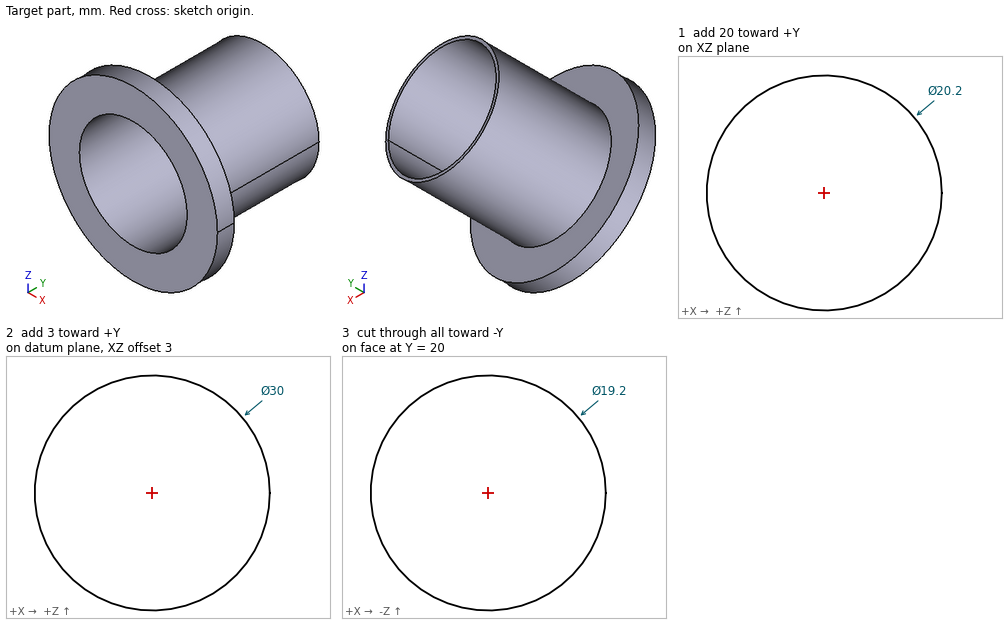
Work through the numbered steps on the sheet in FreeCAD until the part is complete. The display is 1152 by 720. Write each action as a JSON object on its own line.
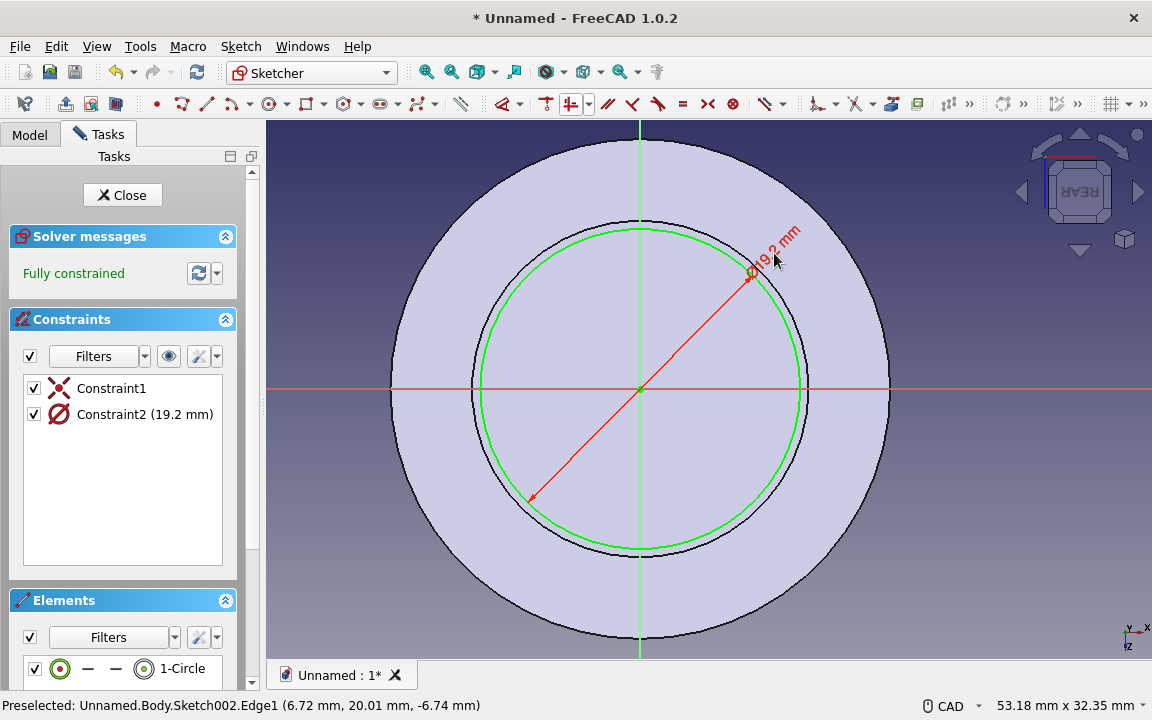
{"action": "left_click", "coordinate": [123, 195]}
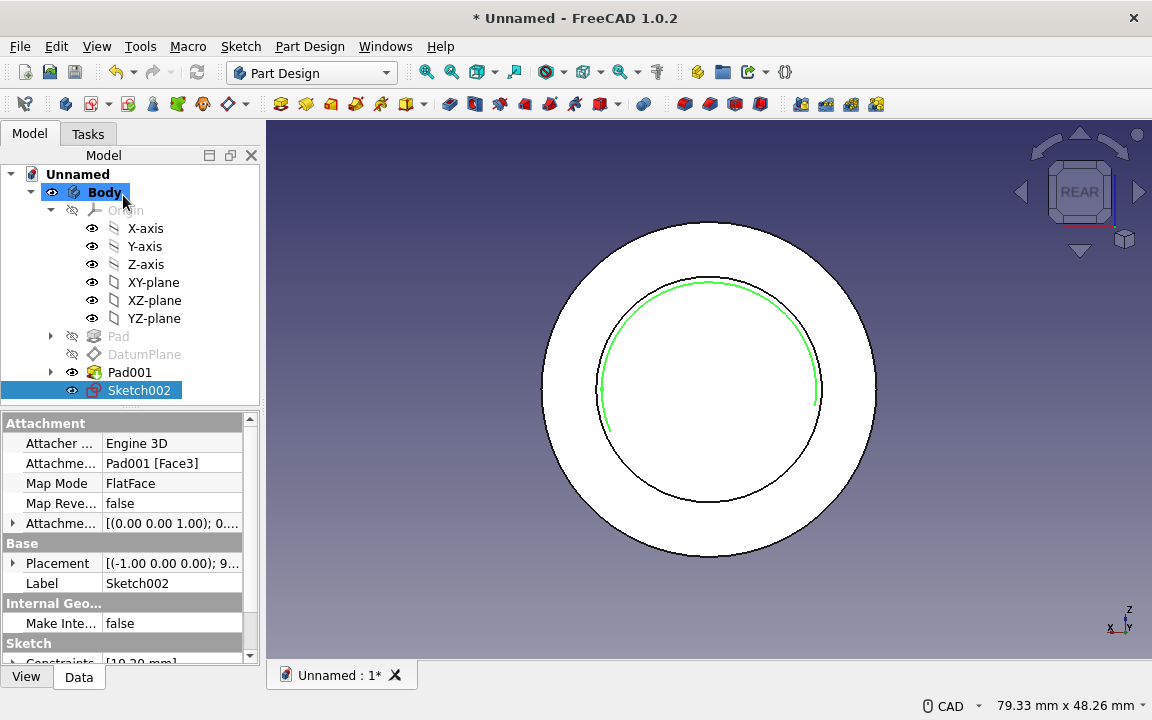
{"action": "left_click", "coordinate": [450, 104]}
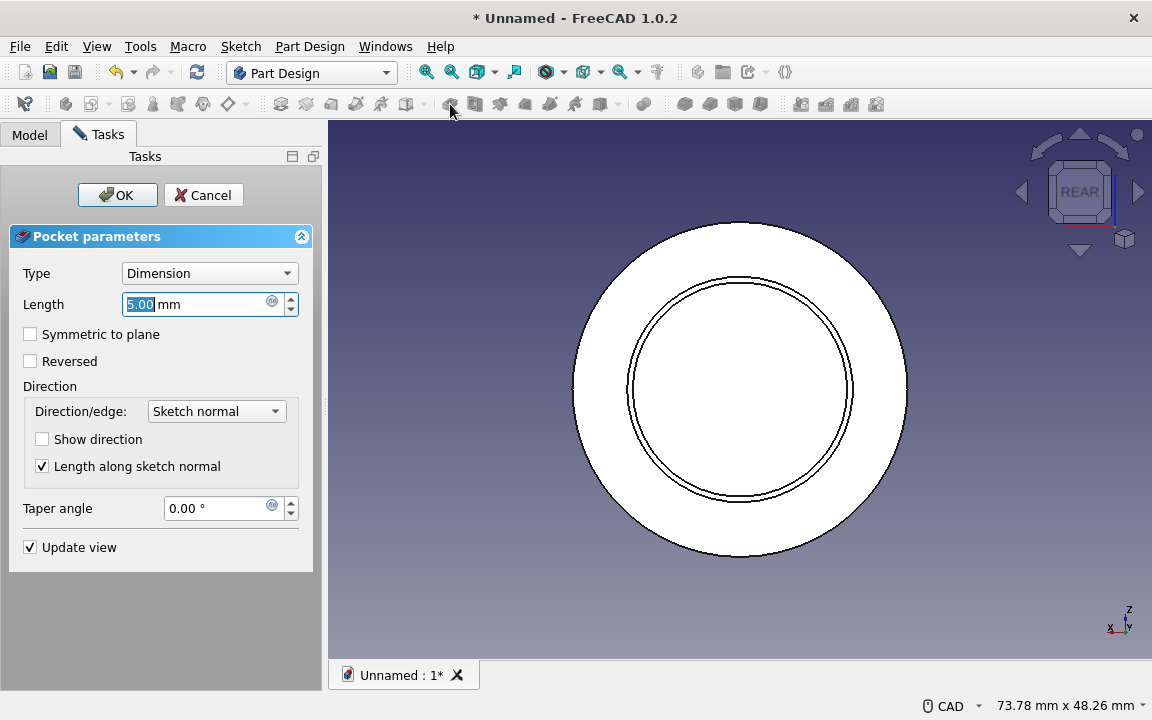
{"action": "left_click", "coordinate": [210, 274]}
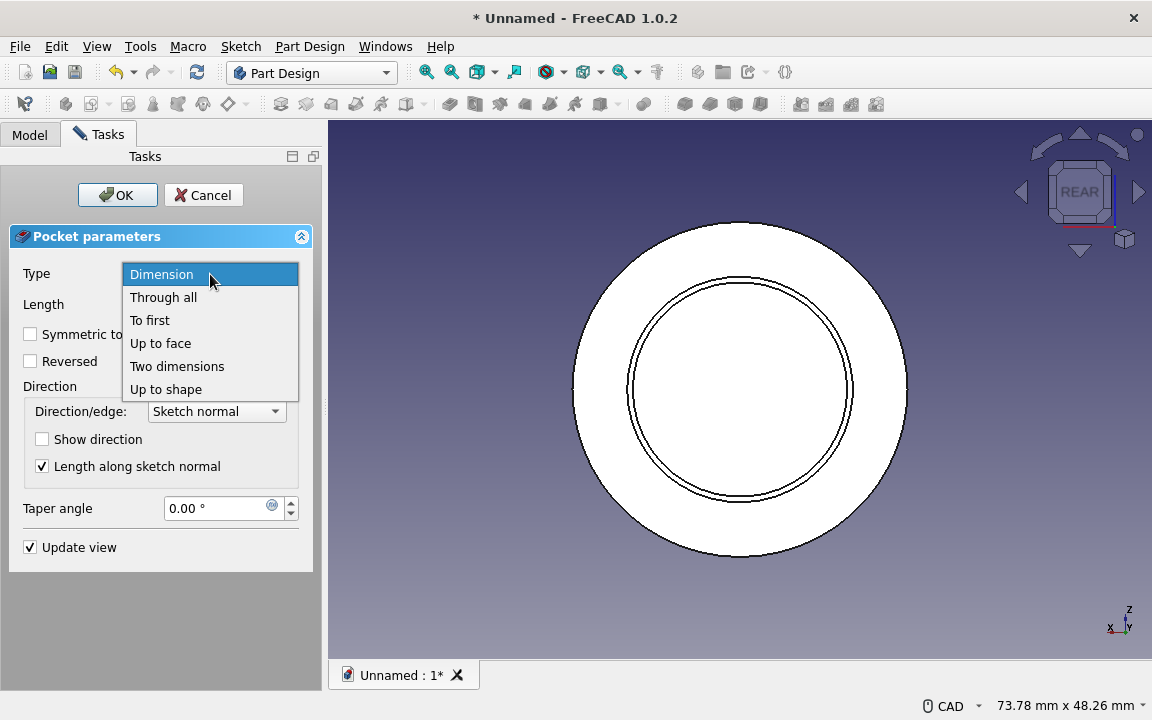
{"action": "left_click", "coordinate": [208, 298]}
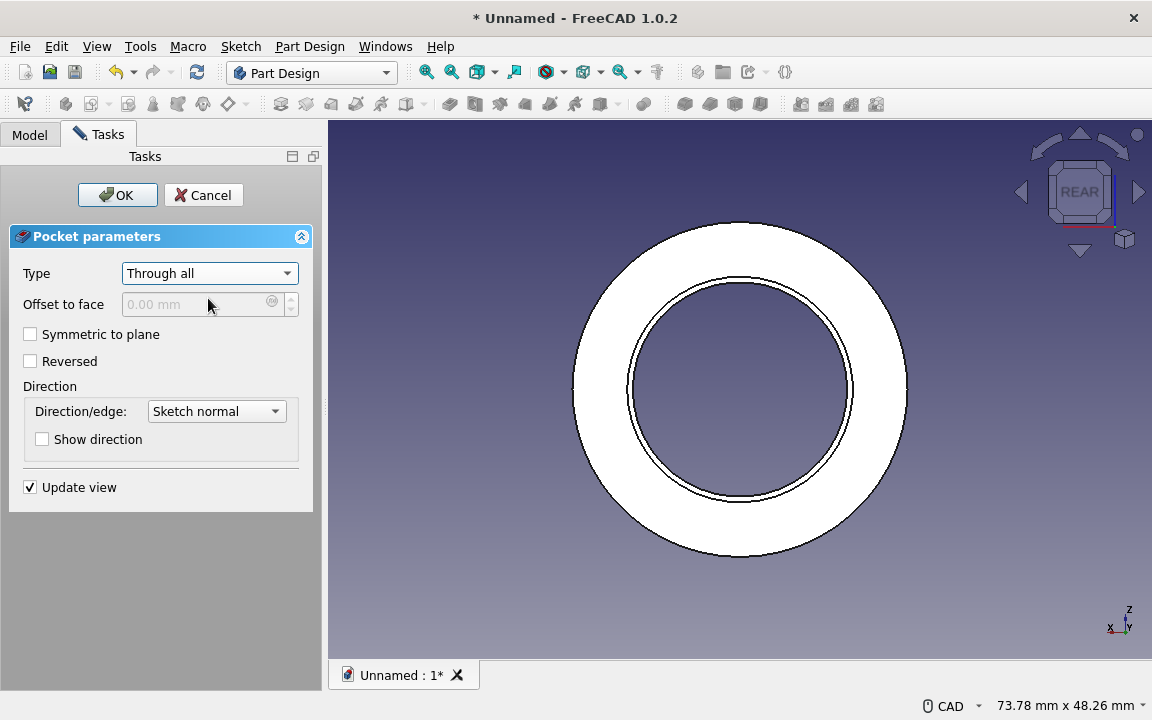
{"action": "left_click", "coordinate": [118, 195]}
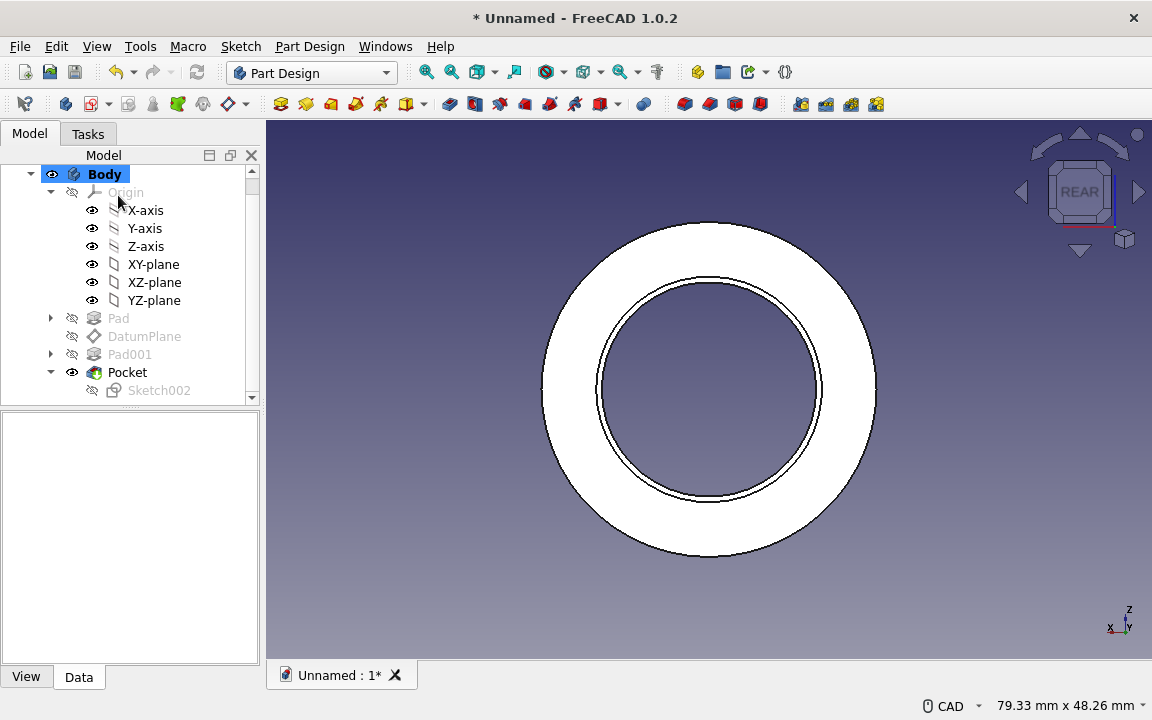
{"action": "key", "text": "0"}